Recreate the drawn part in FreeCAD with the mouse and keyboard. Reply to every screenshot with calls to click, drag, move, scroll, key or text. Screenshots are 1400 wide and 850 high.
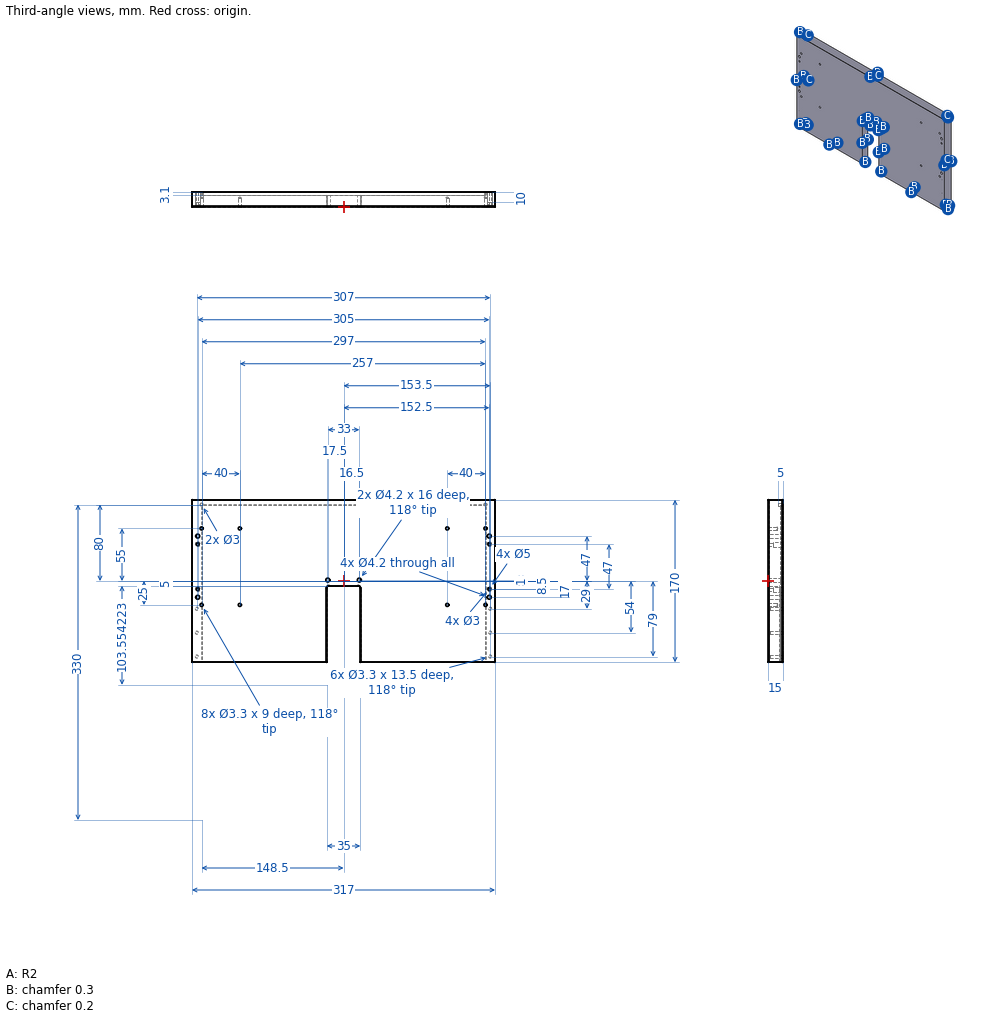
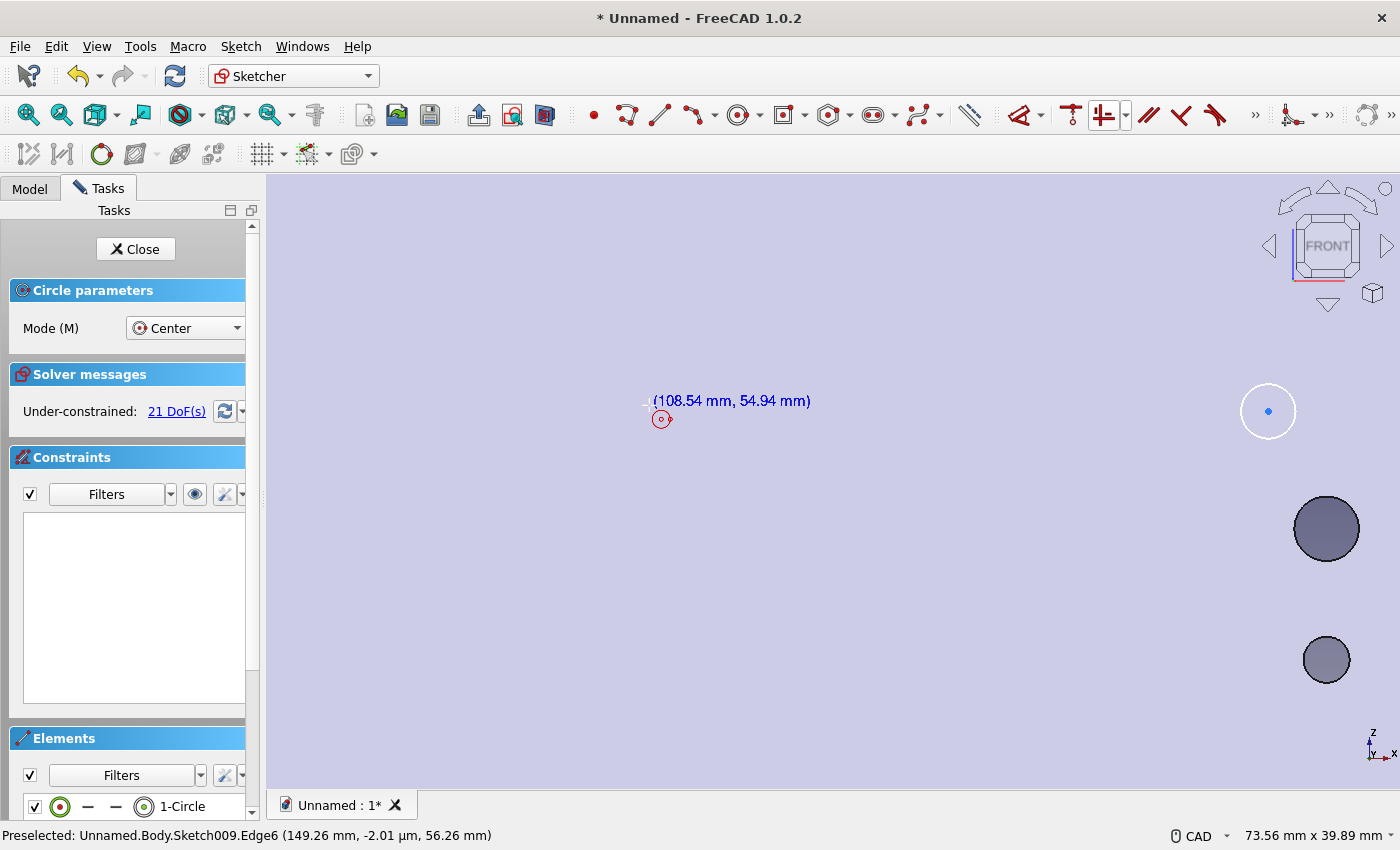
scroll(1044, 397, down, 10)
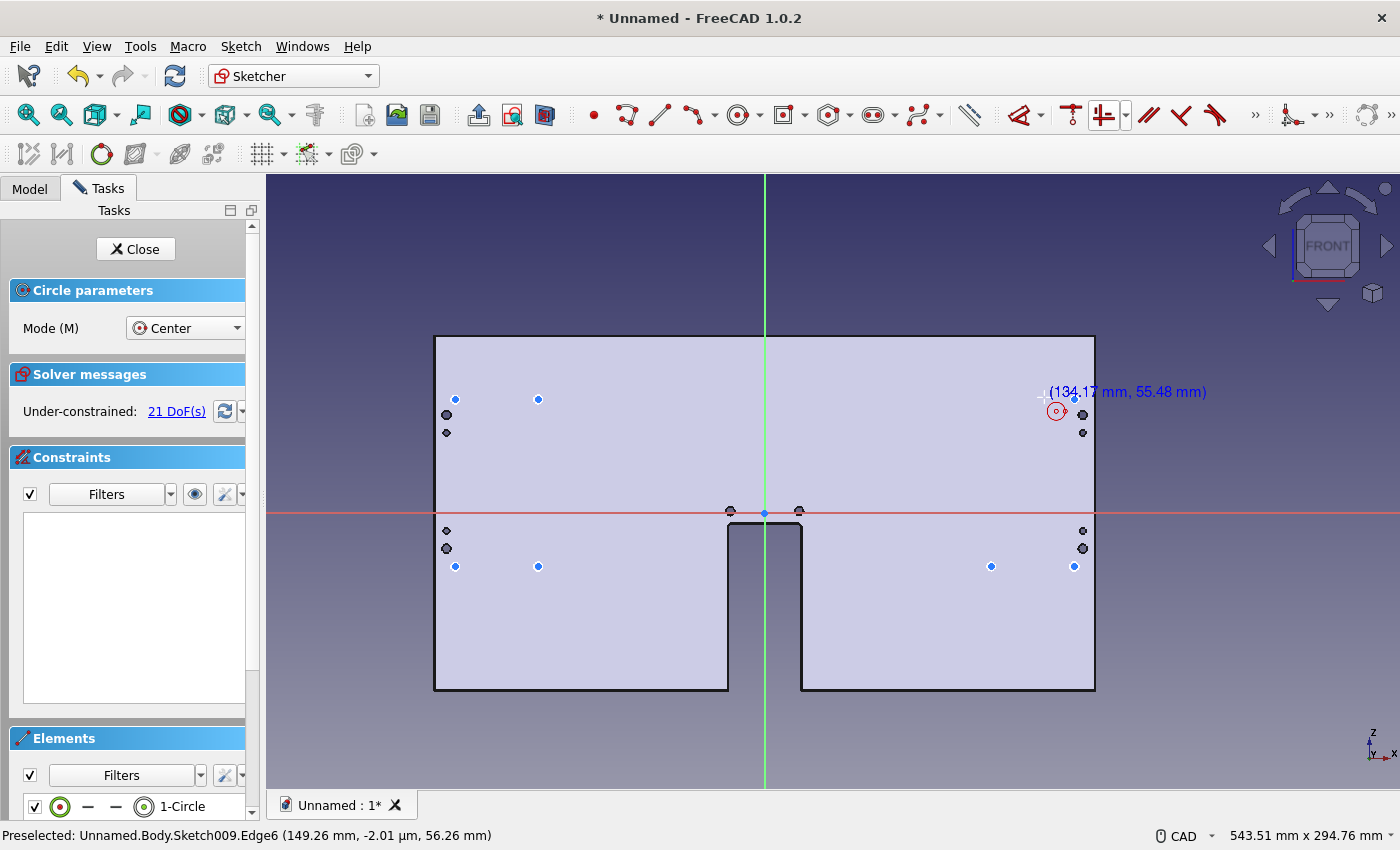
click(991, 398)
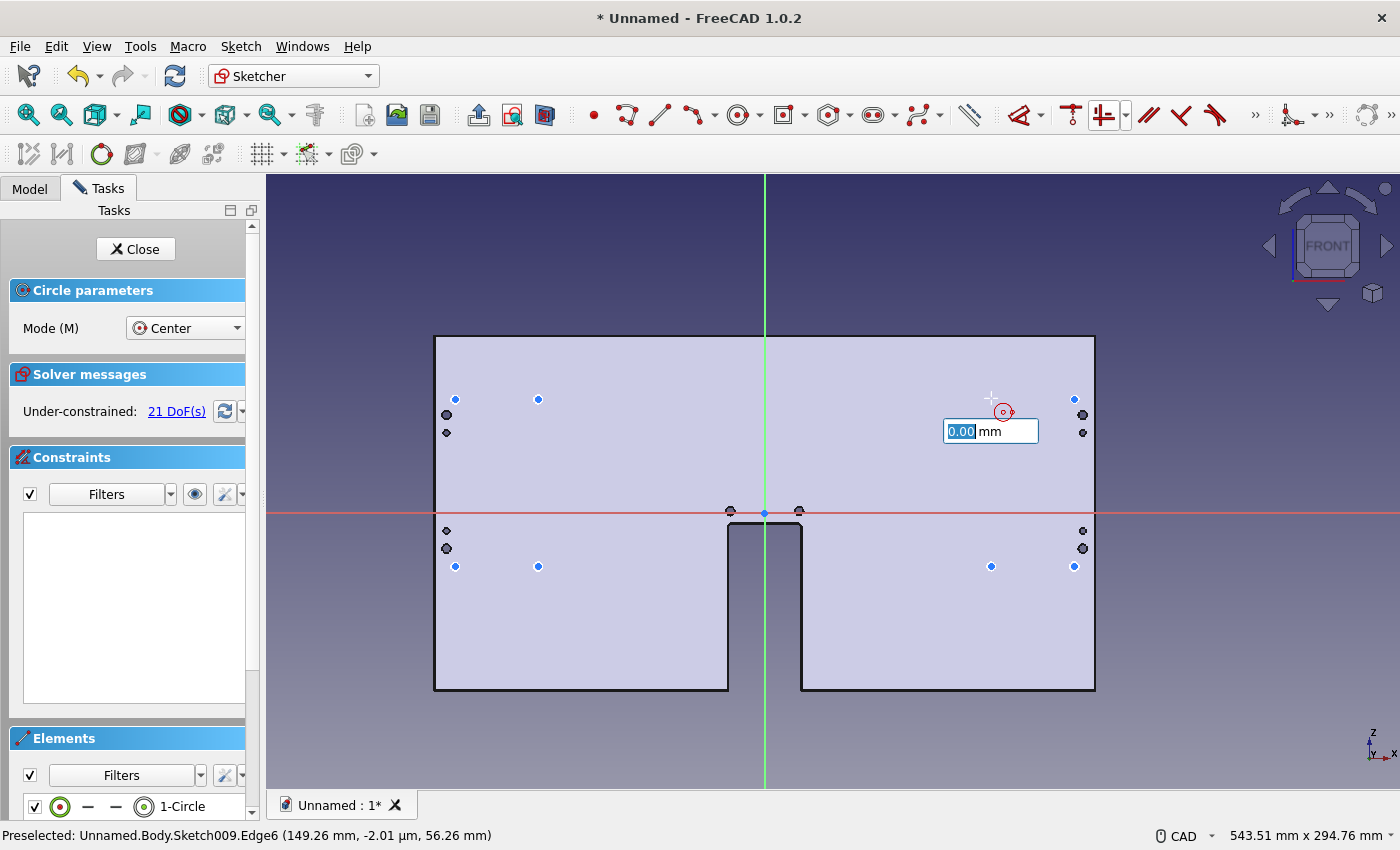
scroll(993, 396, up, 8)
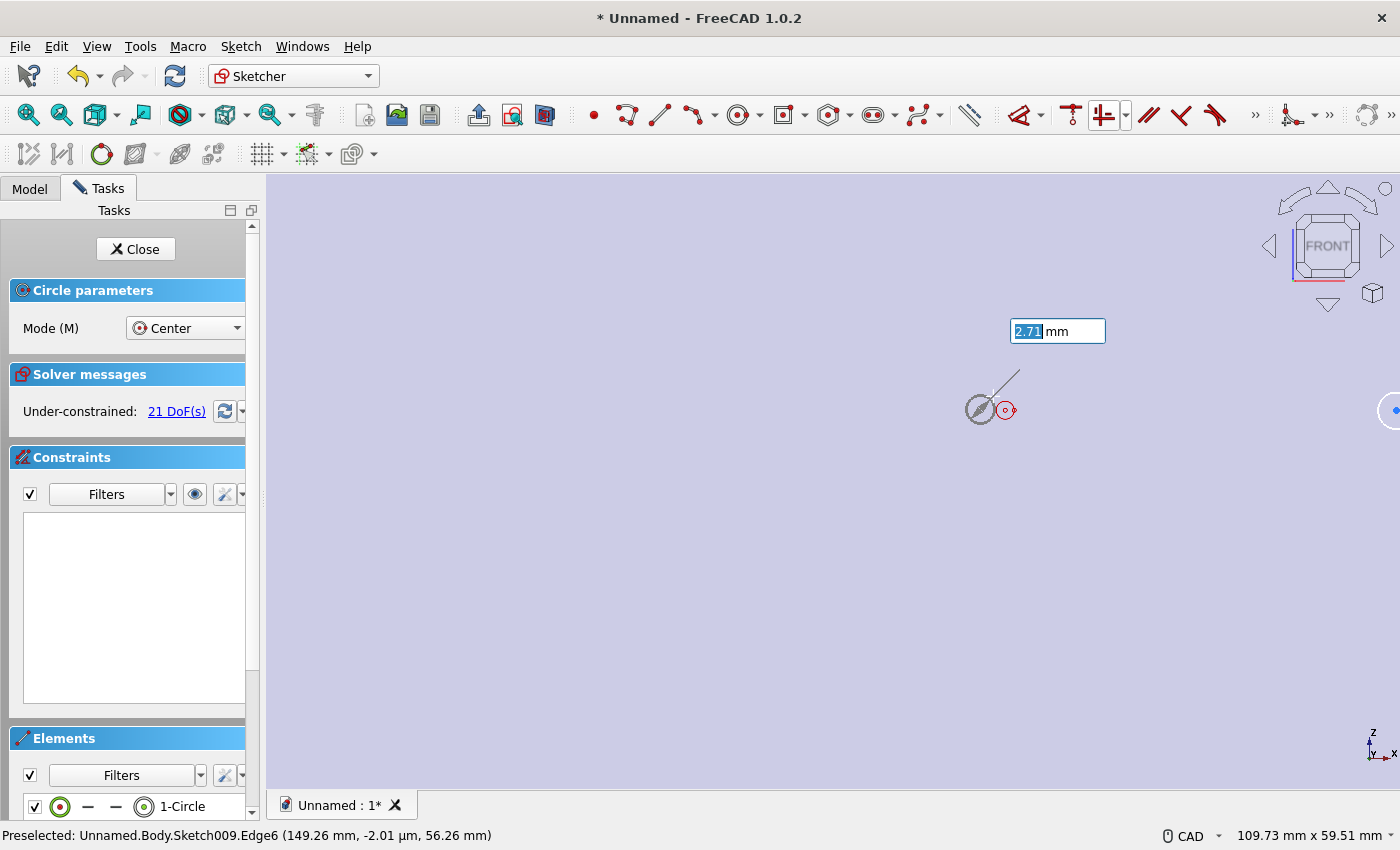
click(993, 395)
key(Escape)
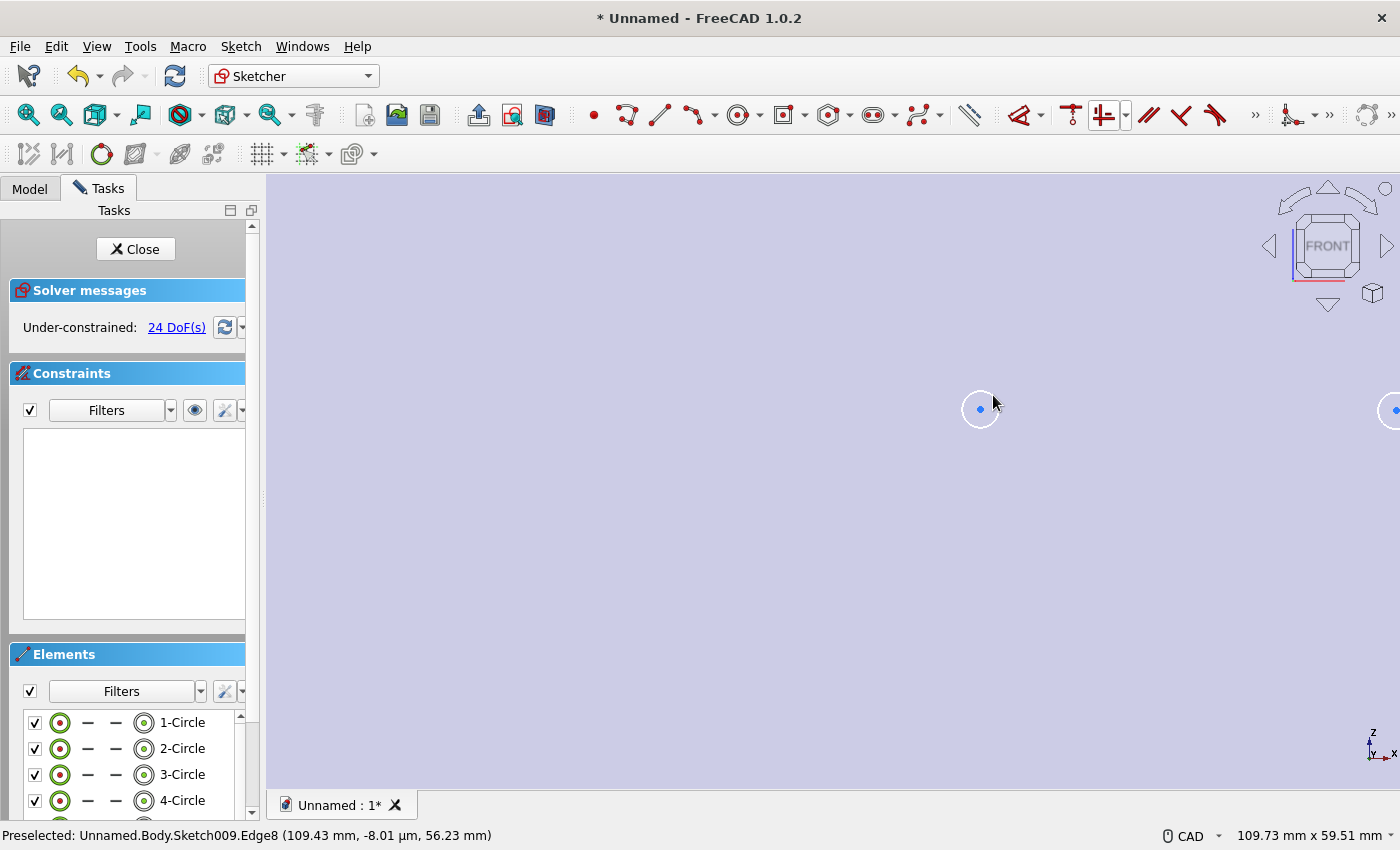
scroll(993, 396, down, 8)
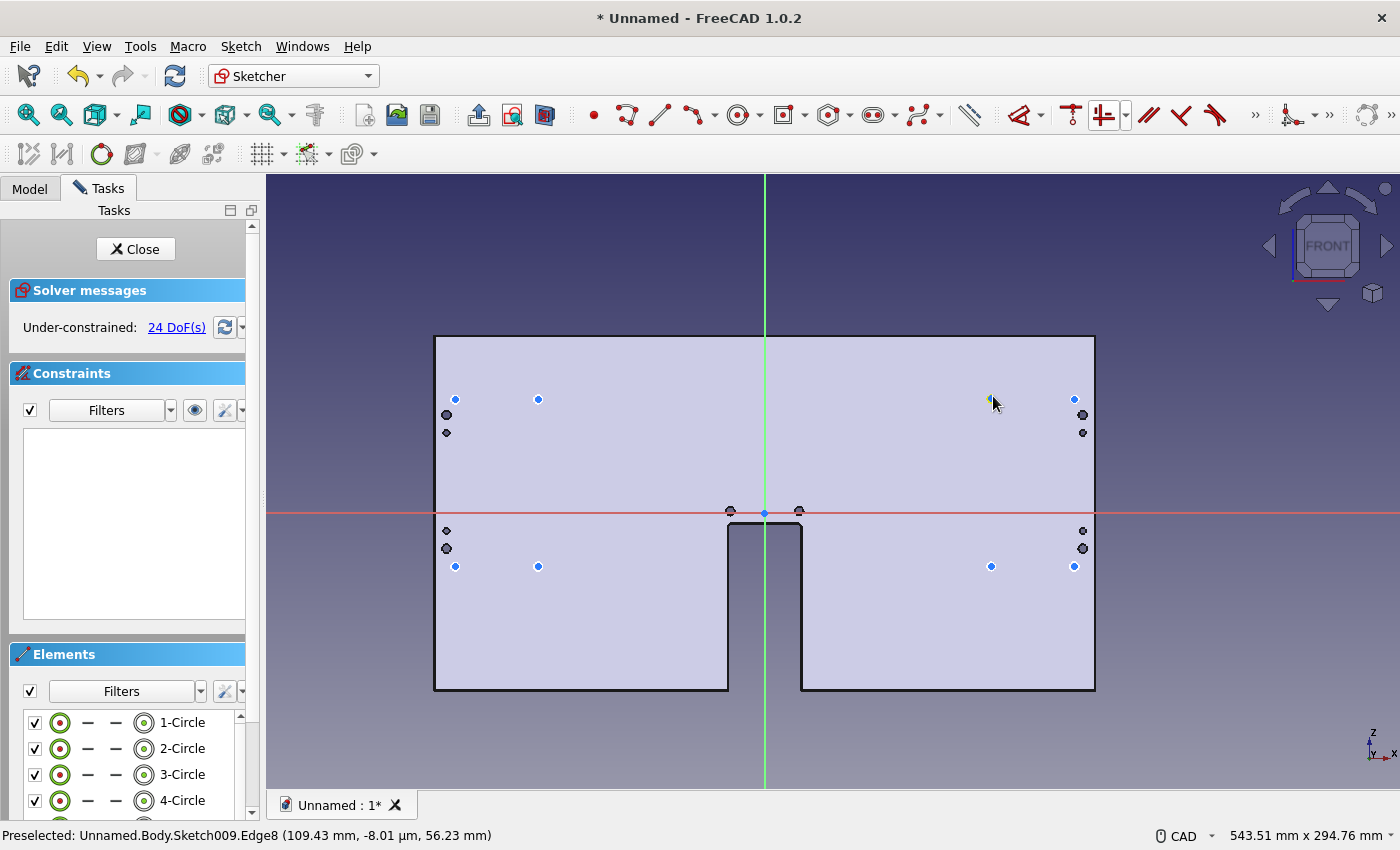
scroll(458, 564, up, 7)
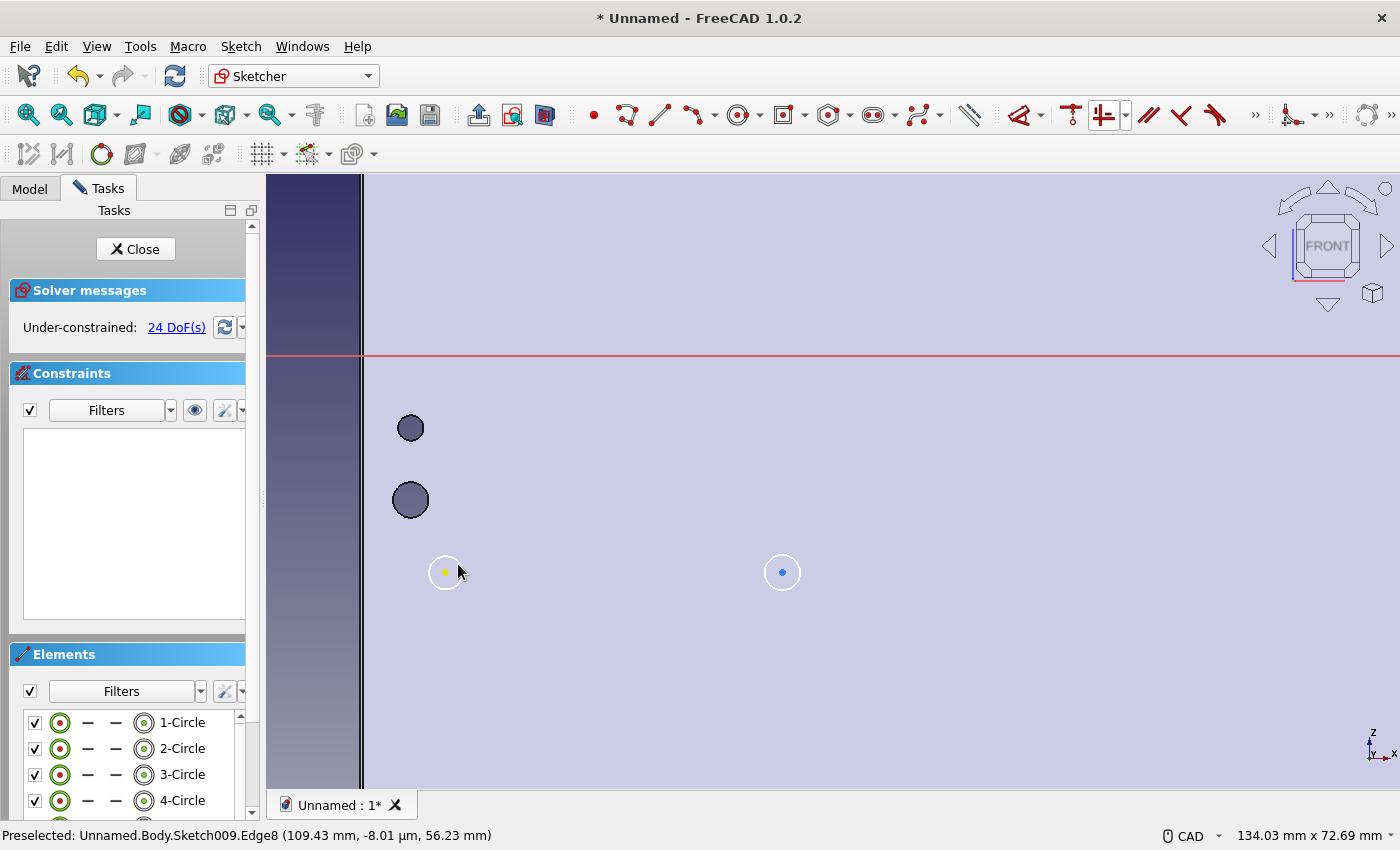
click(457, 561)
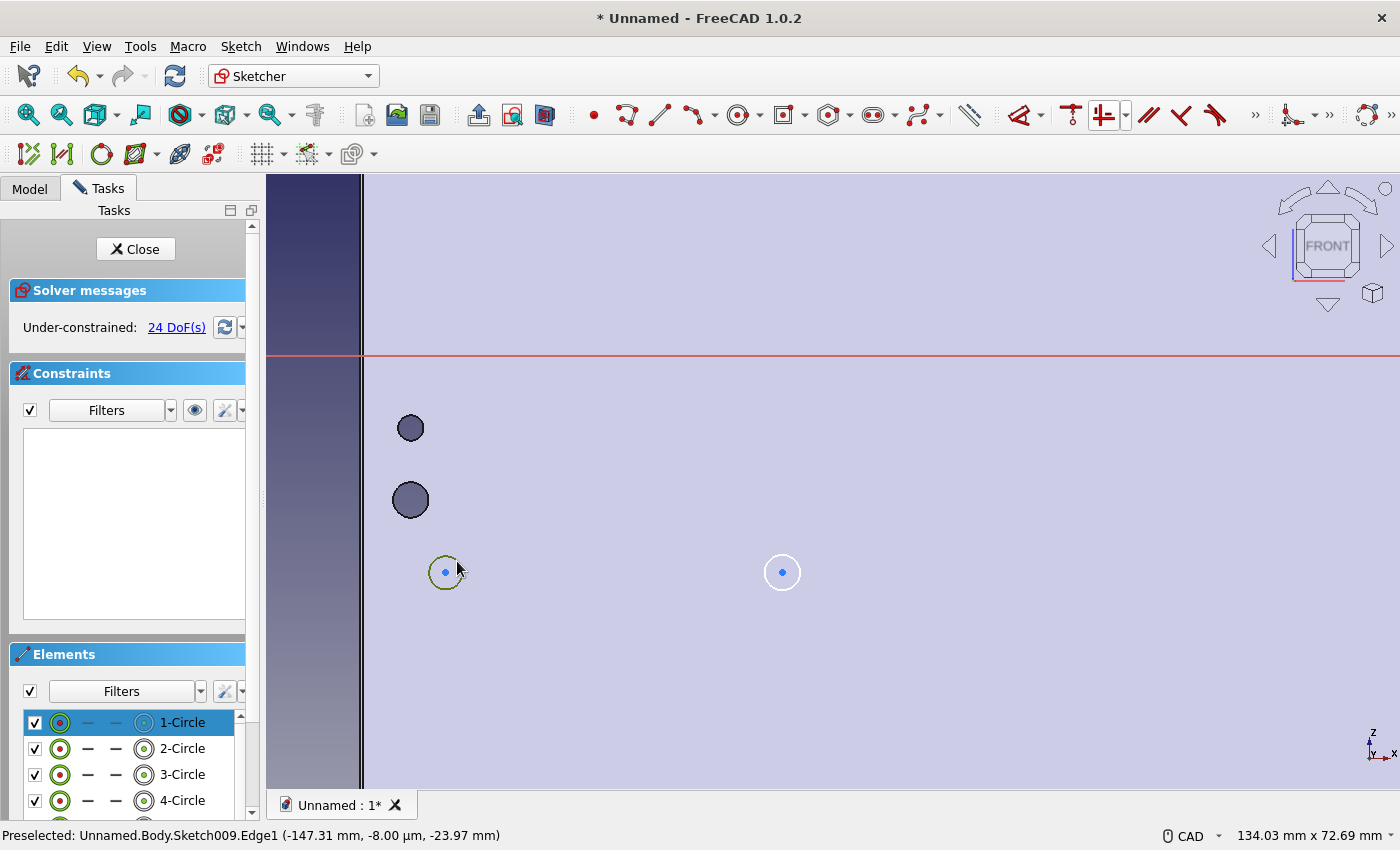
scroll(458, 564, down, 7)